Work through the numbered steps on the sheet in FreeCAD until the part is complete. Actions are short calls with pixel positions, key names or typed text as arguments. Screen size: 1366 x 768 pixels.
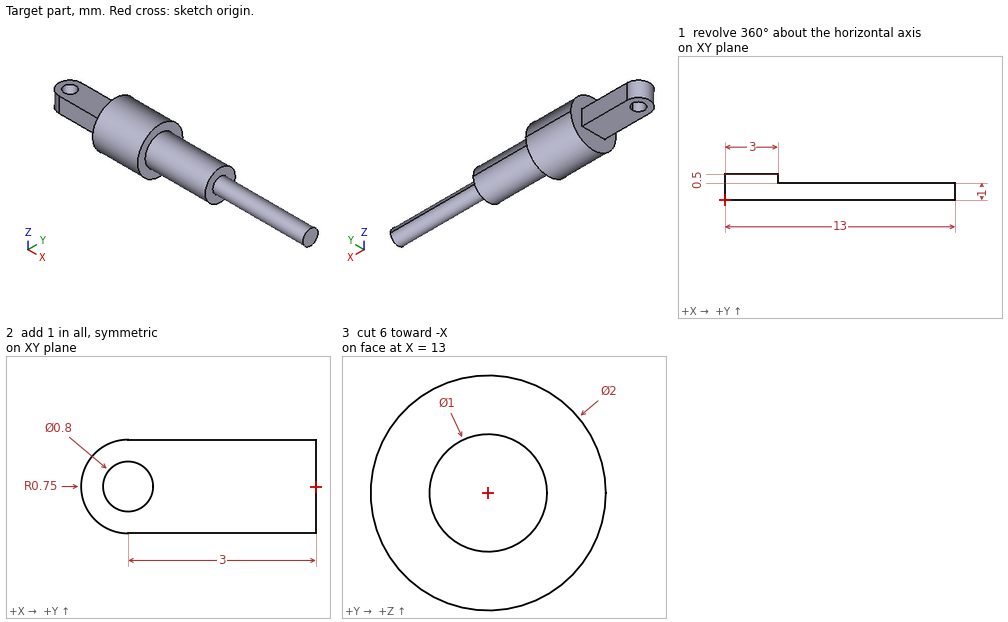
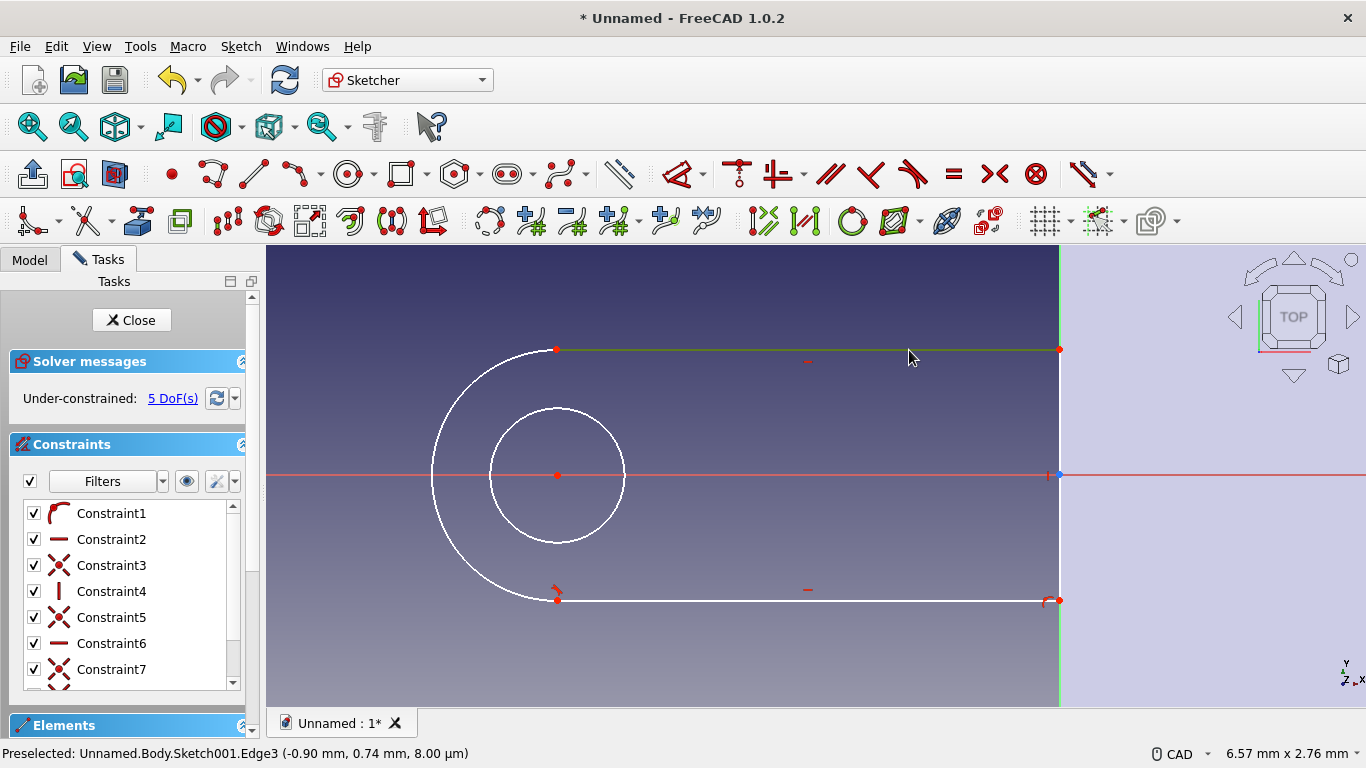
click(456, 402)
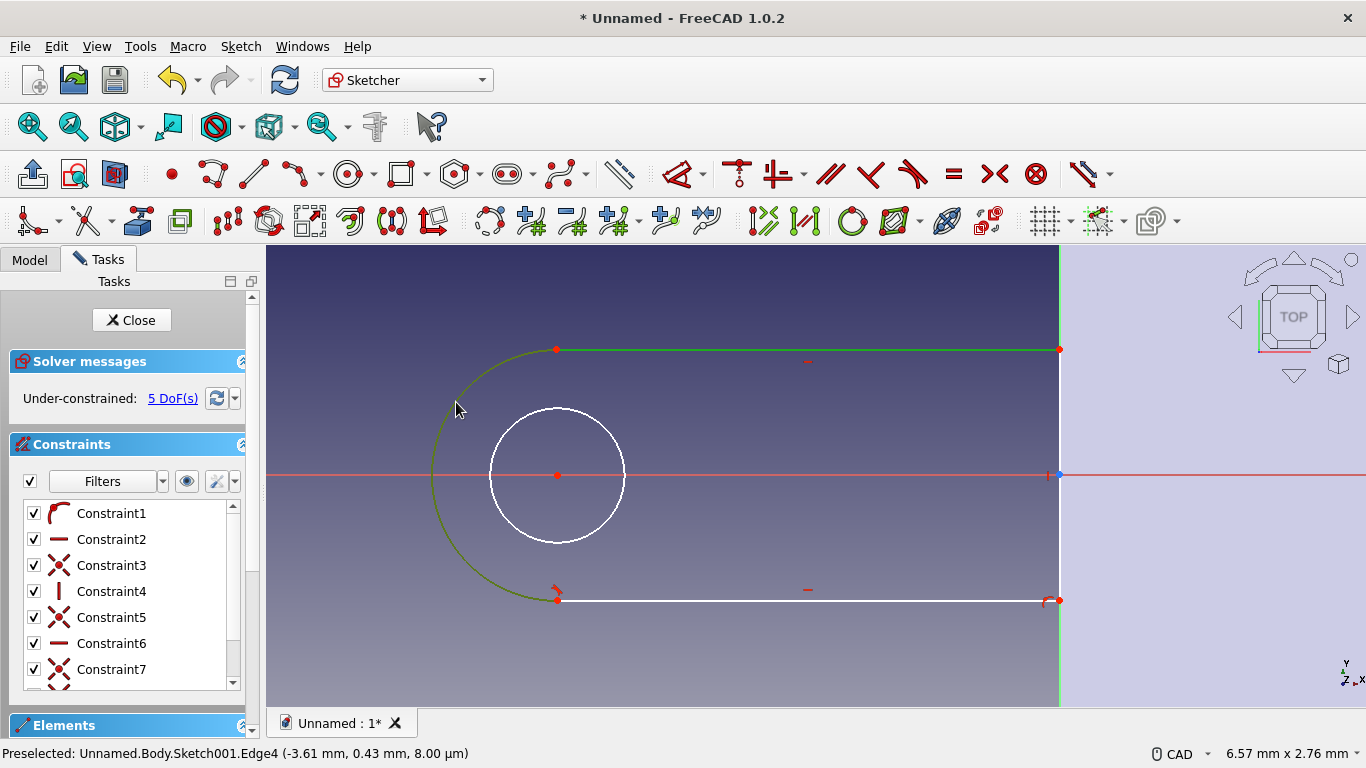
key(t)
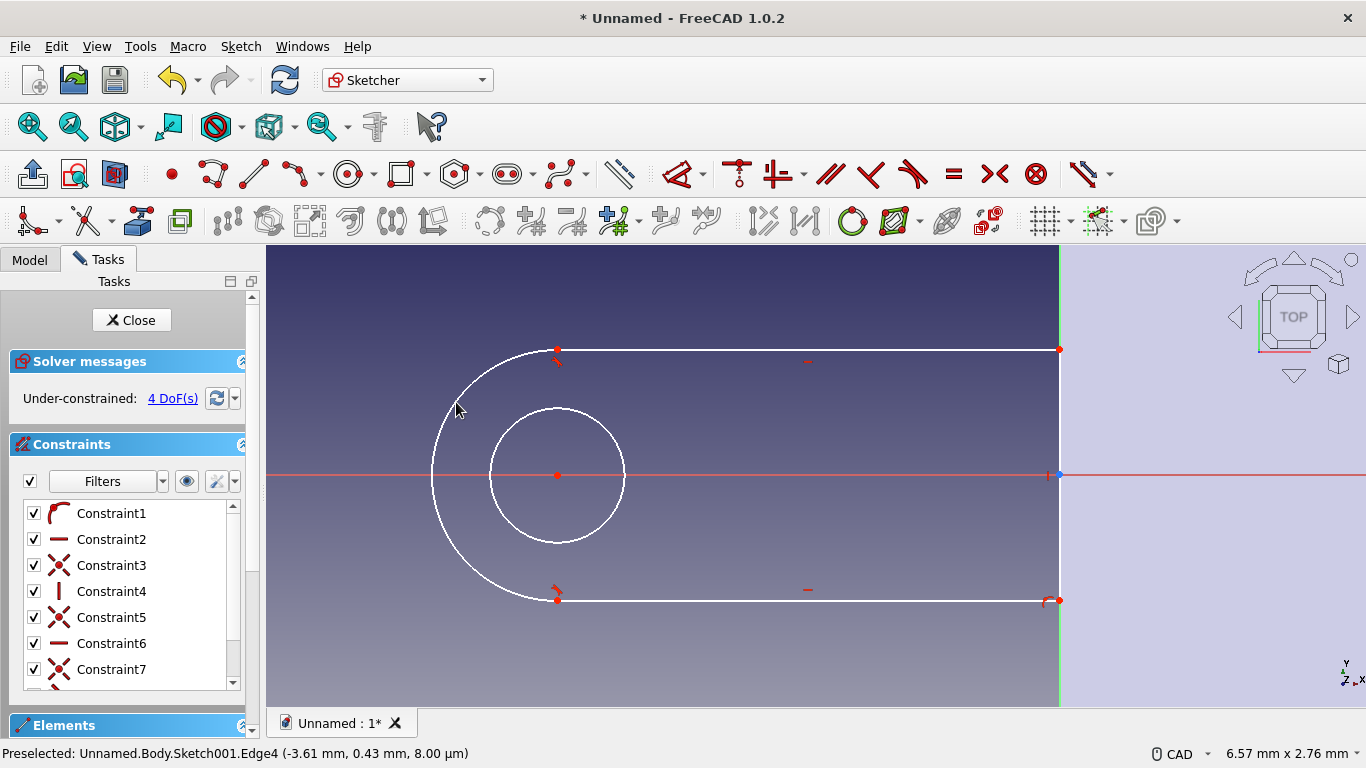
click(557, 476)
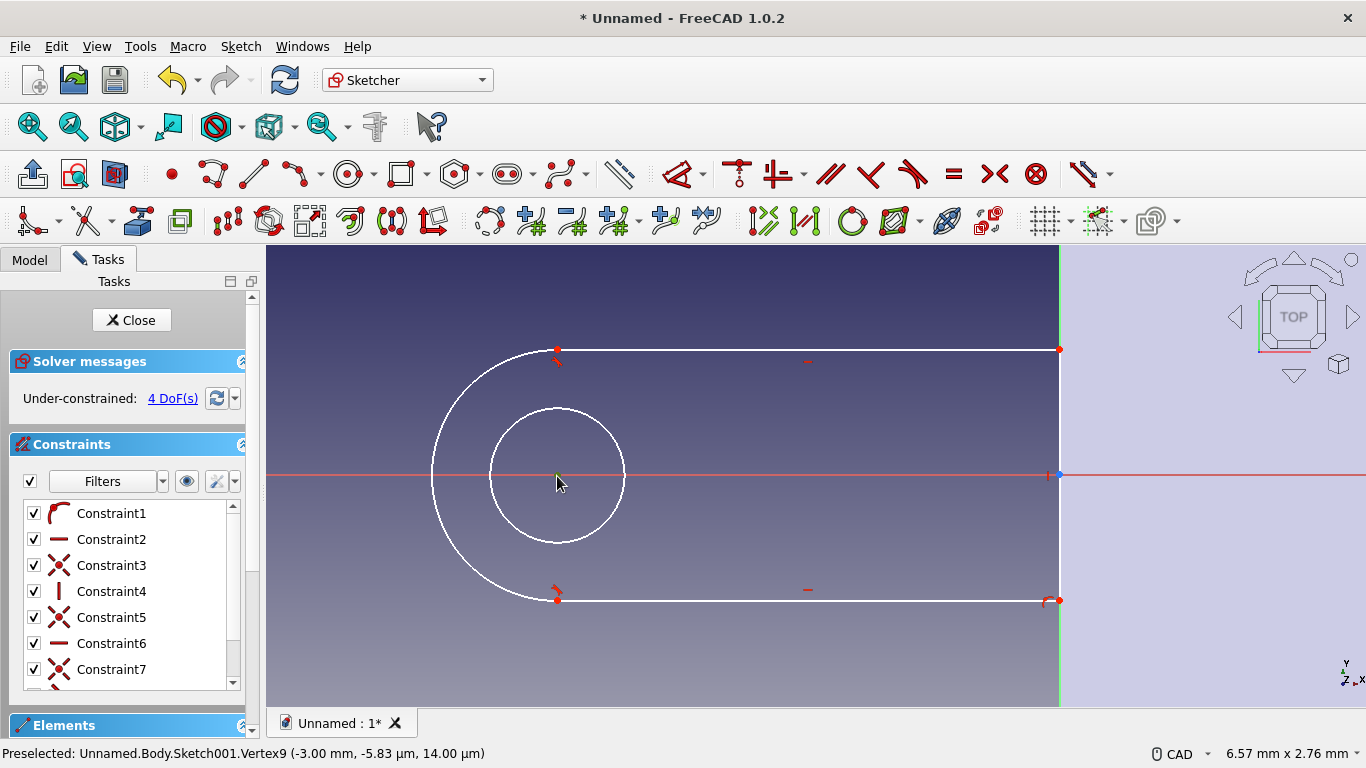
click(359, 475)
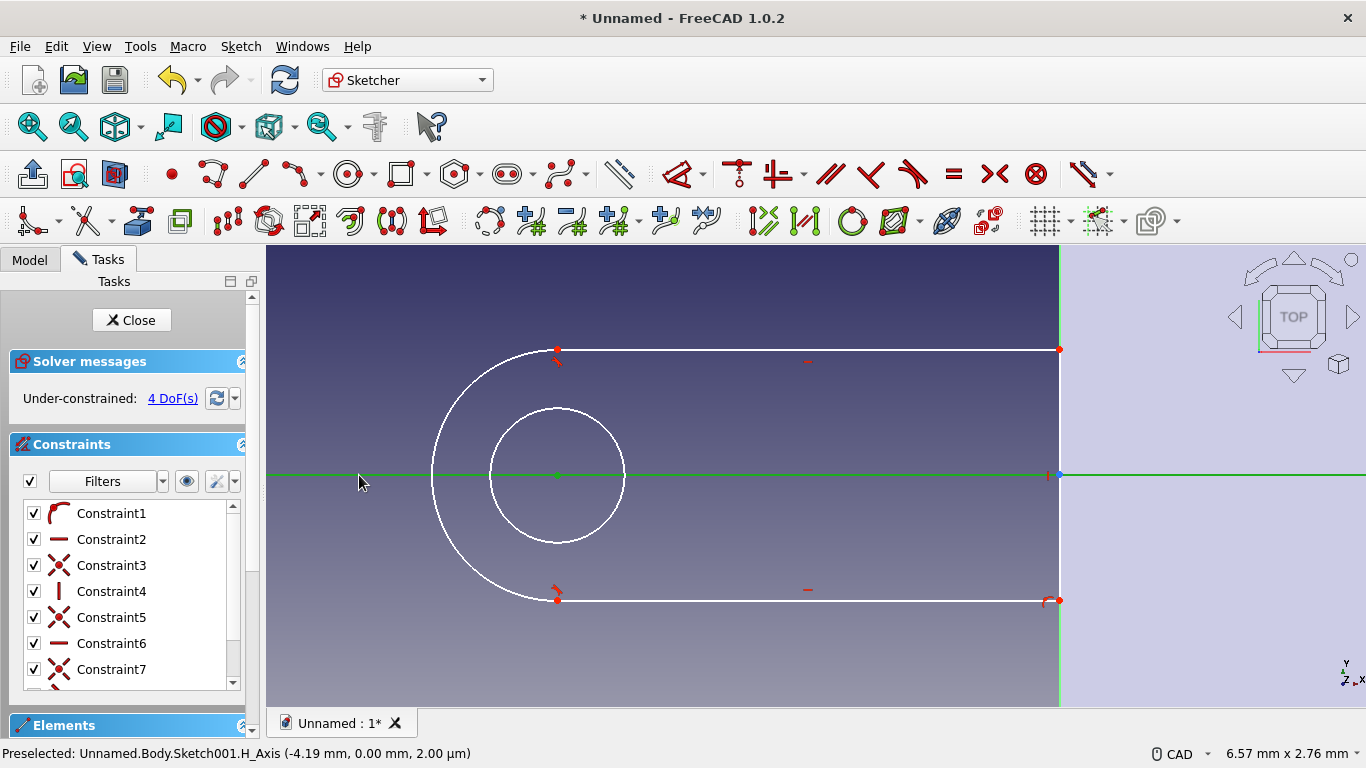
key(c)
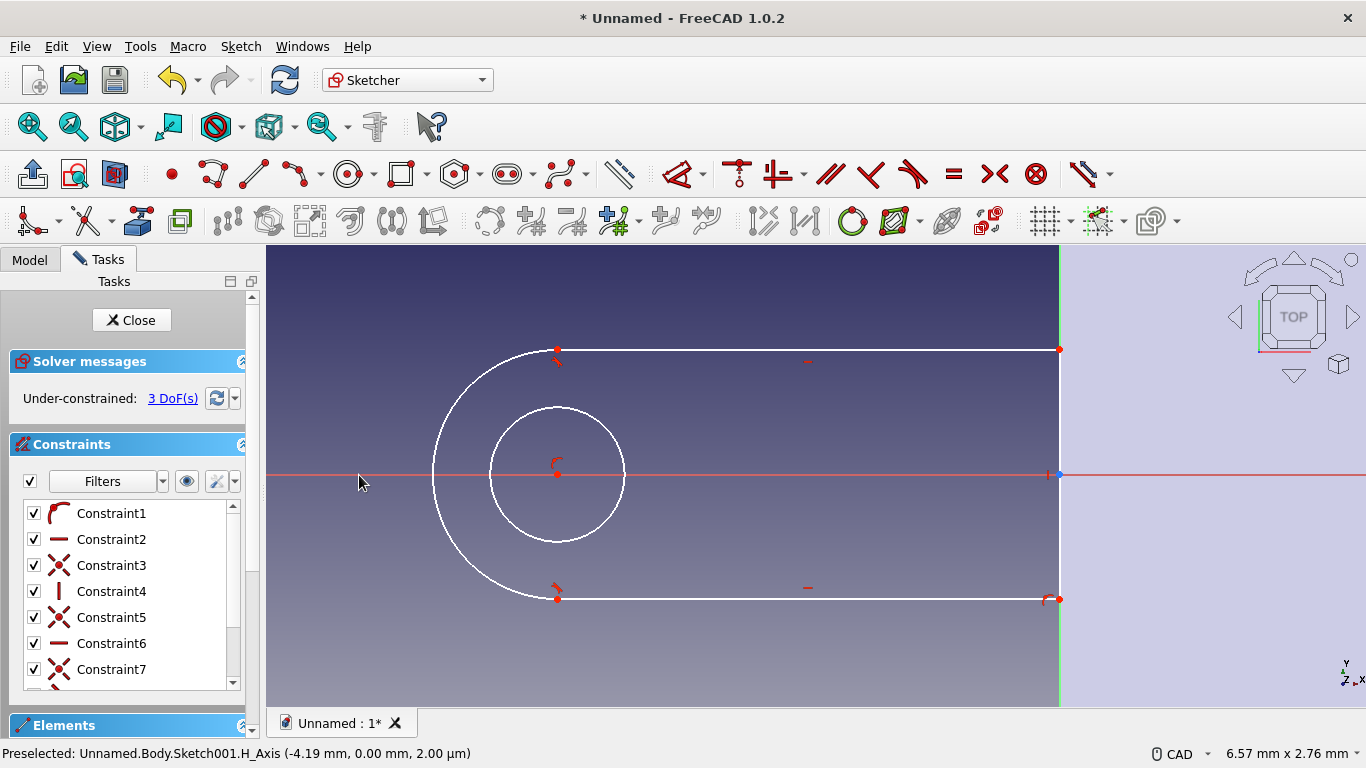
key(d)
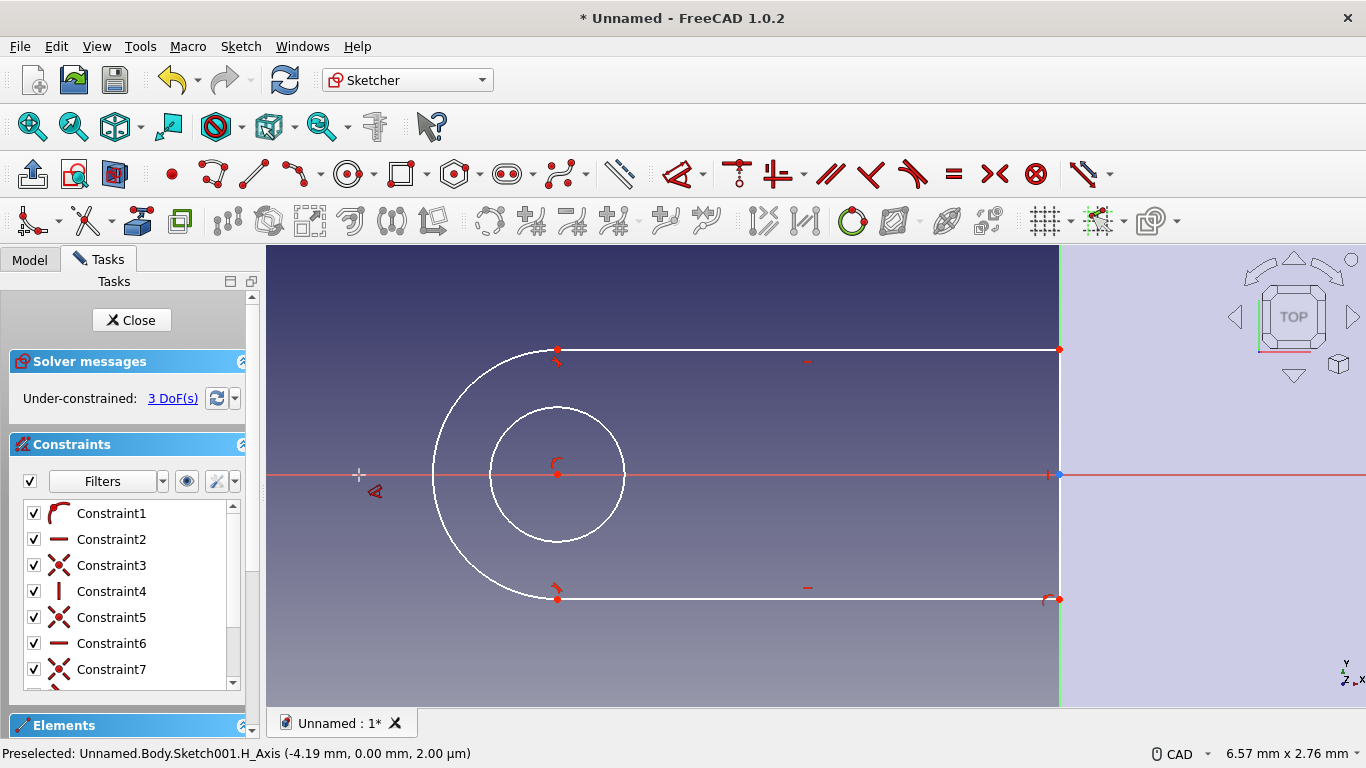
click(457, 401)
click(431, 382)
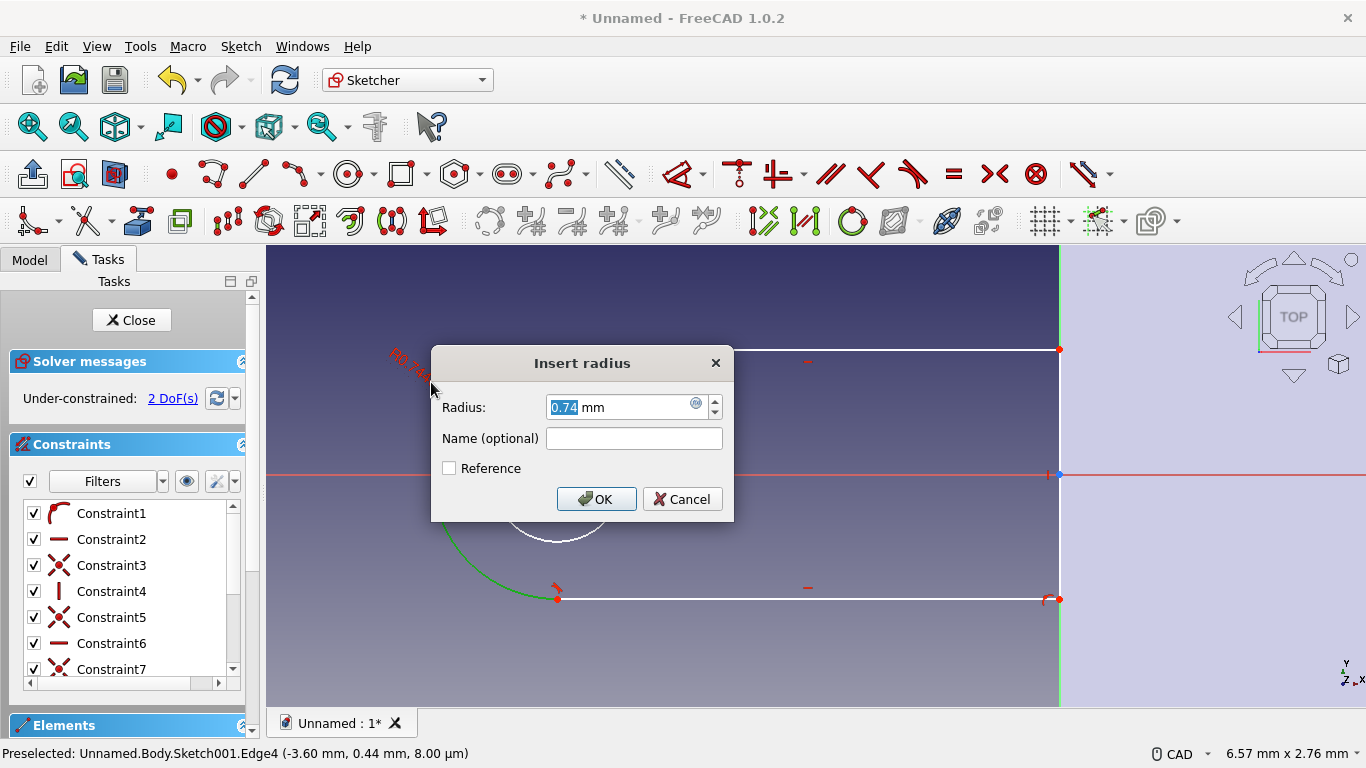
text(0.75)
key(Return)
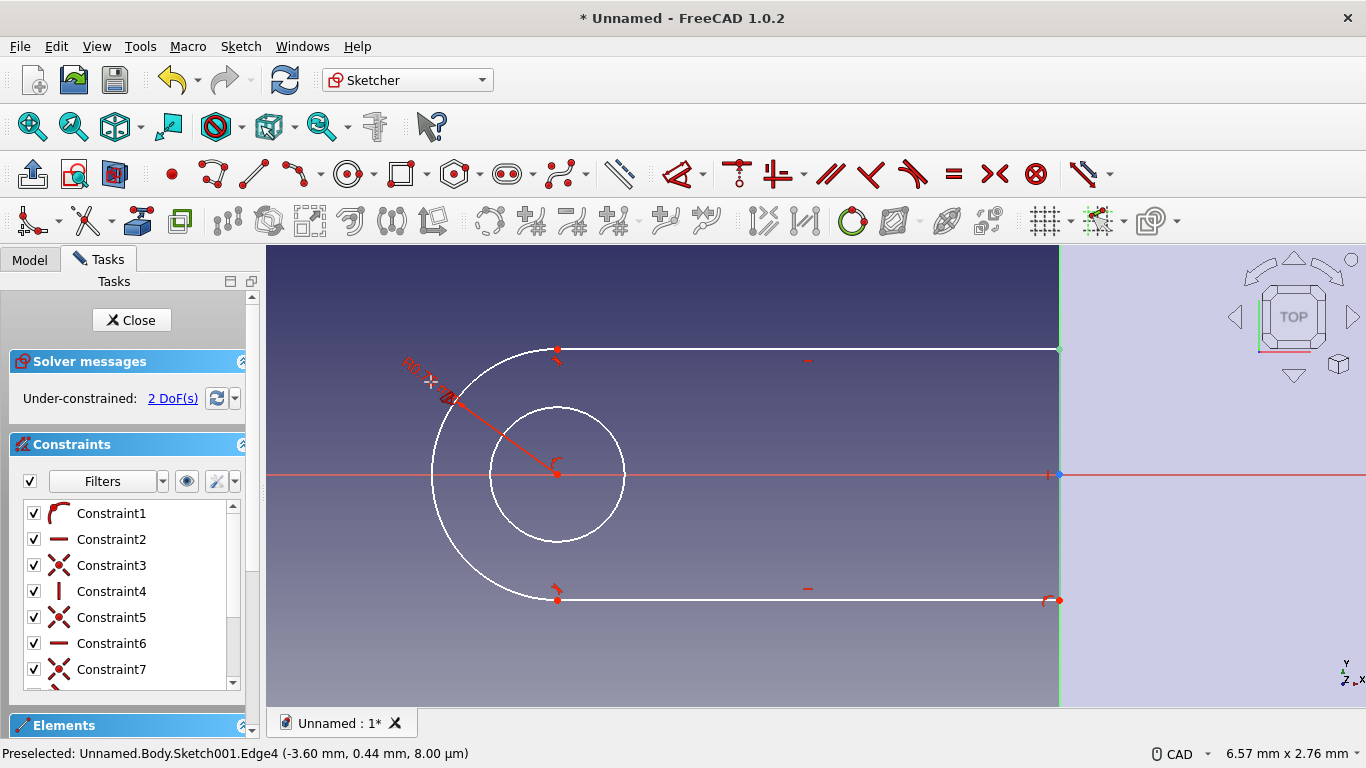
click(605, 427)
click(628, 404)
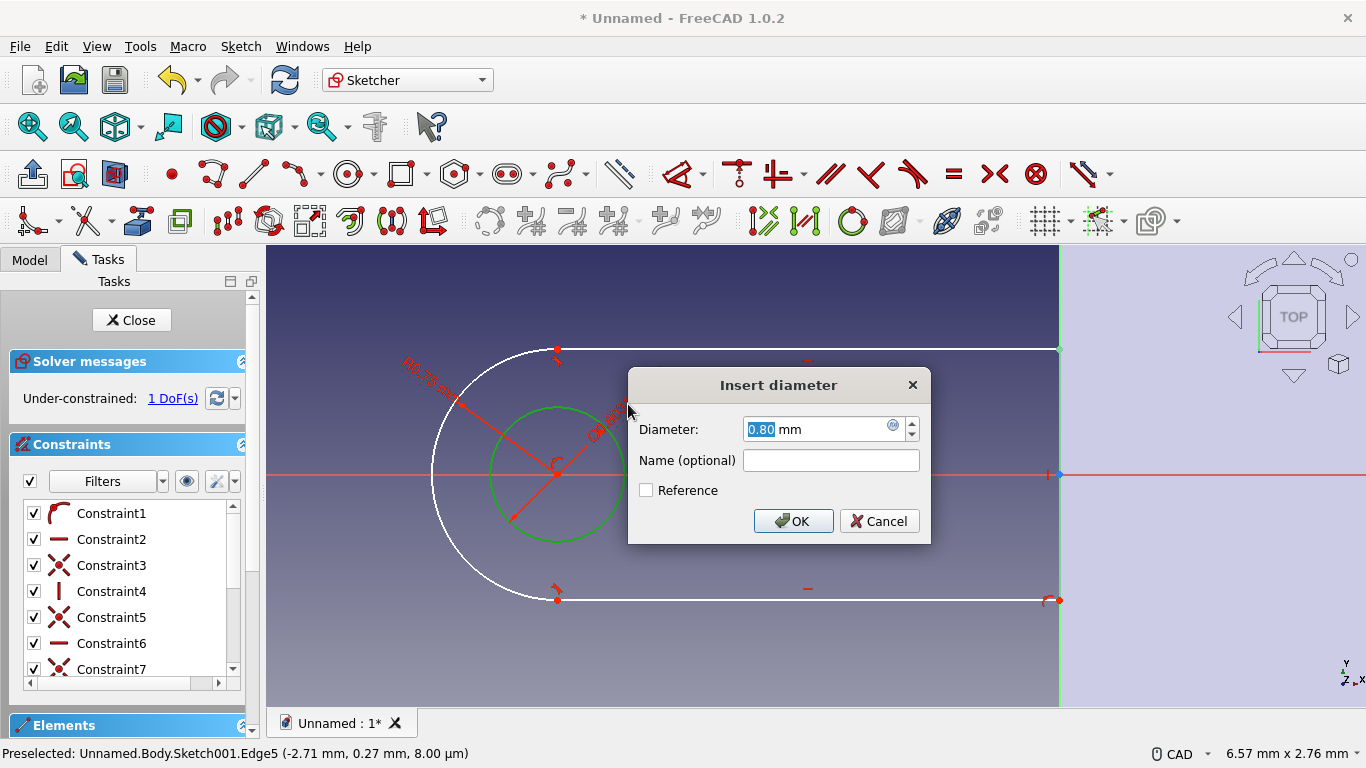
text(0.8)
key(Return)